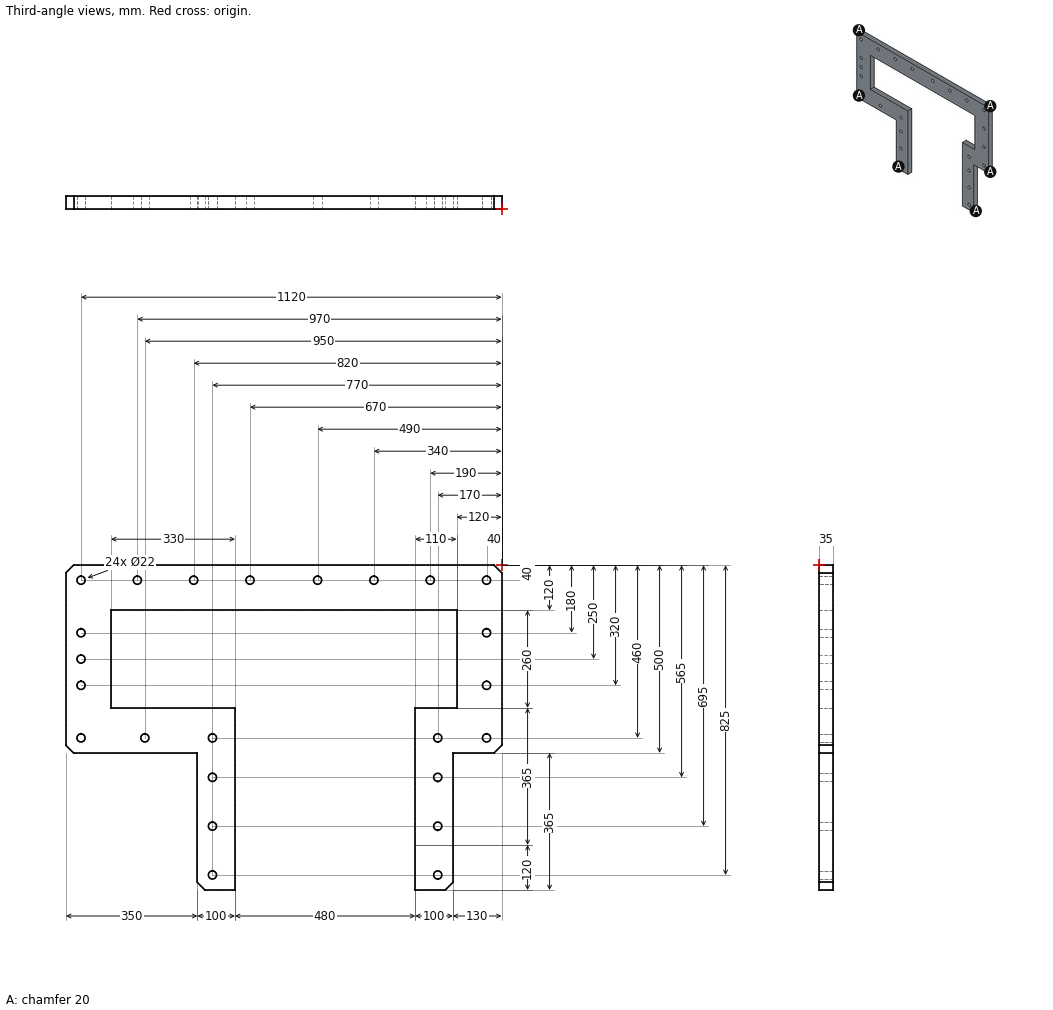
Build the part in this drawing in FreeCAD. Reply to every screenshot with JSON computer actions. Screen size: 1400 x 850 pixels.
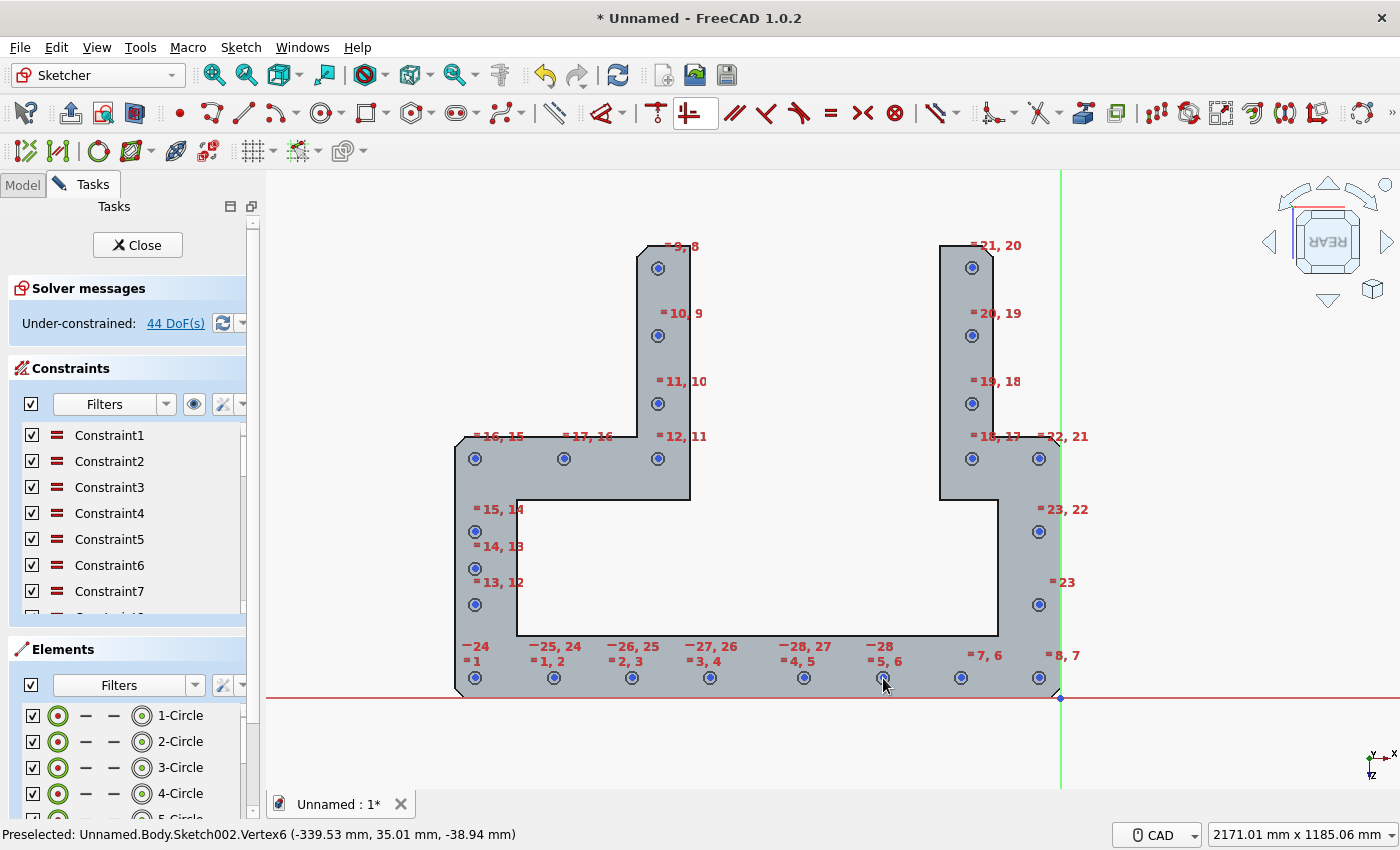
{"action": "left_click", "coordinate": [883, 678]}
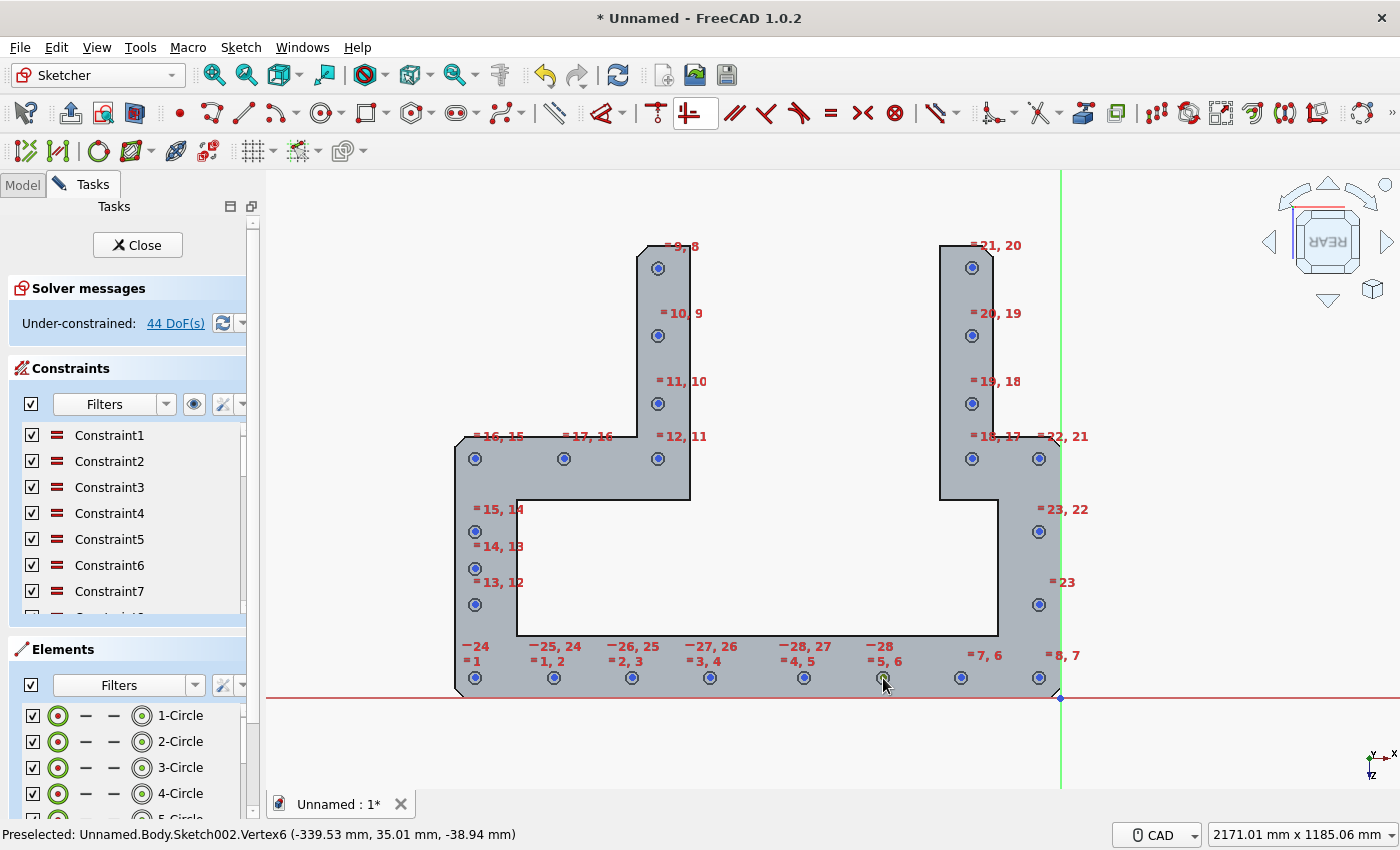
{"action": "left_click", "coordinate": [961, 678]}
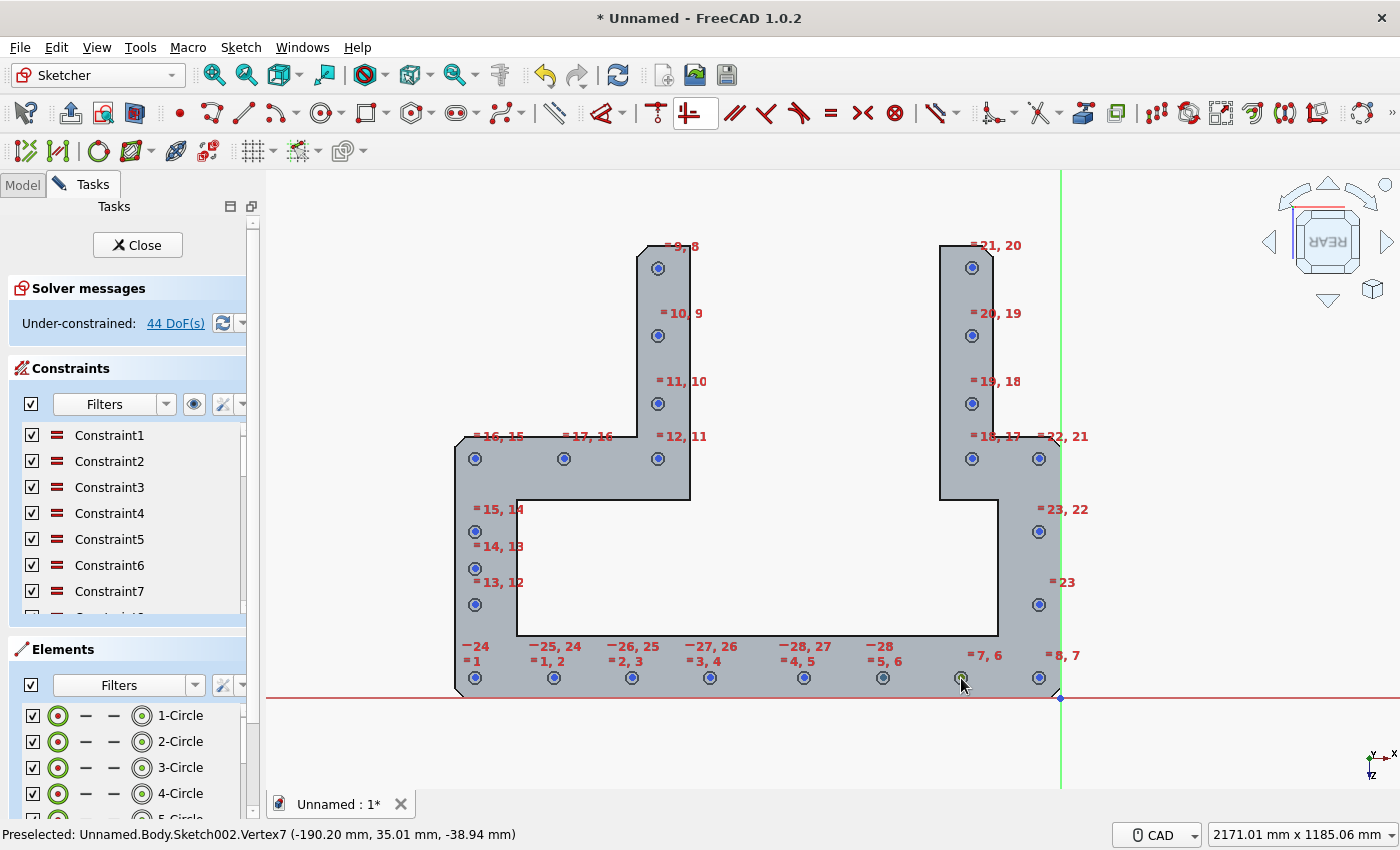
{"action": "left_click", "coordinate": [712, 114]}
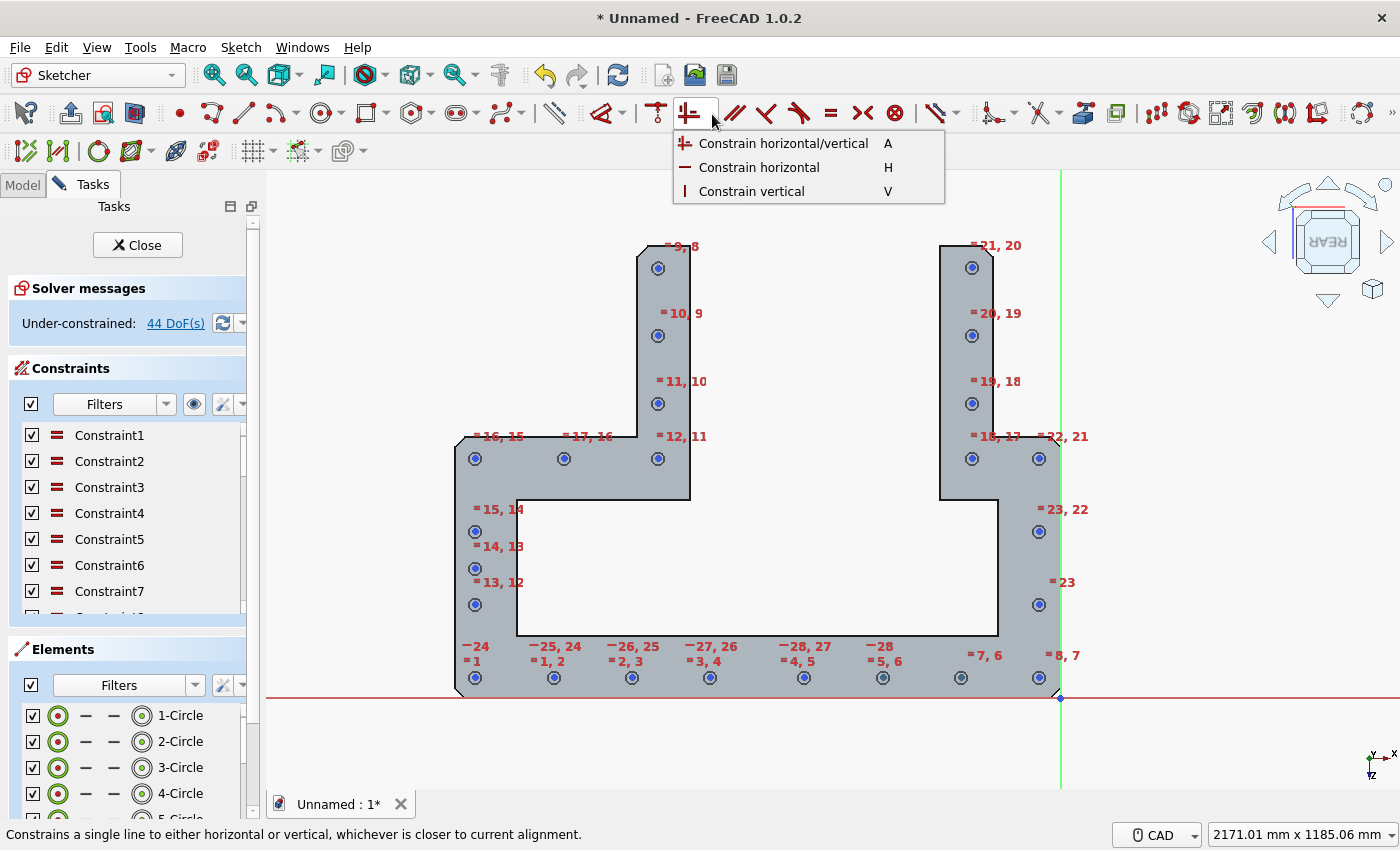
{"action": "left_click", "coordinate": [809, 167]}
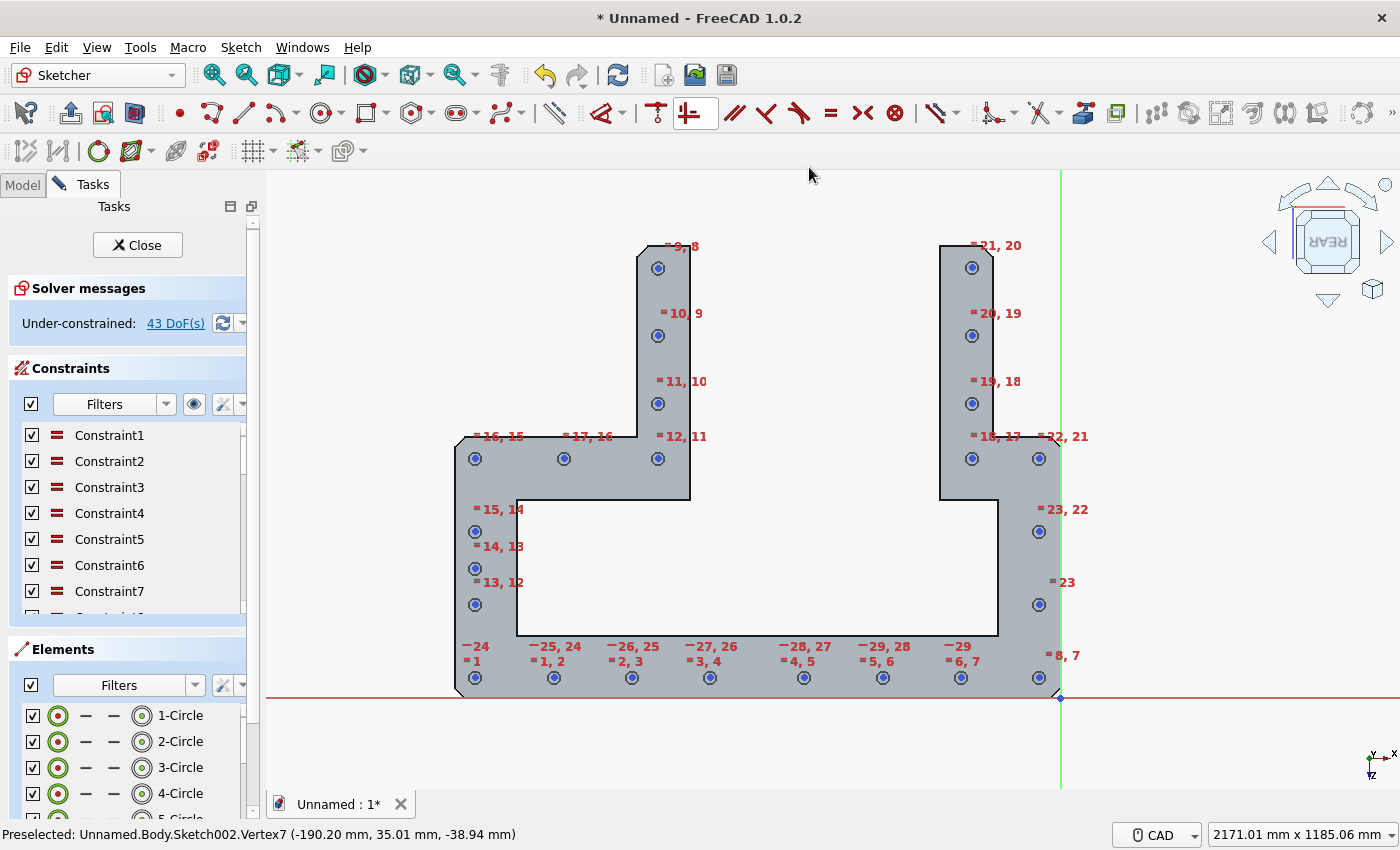
{"action": "left_click", "coordinate": [961, 678]}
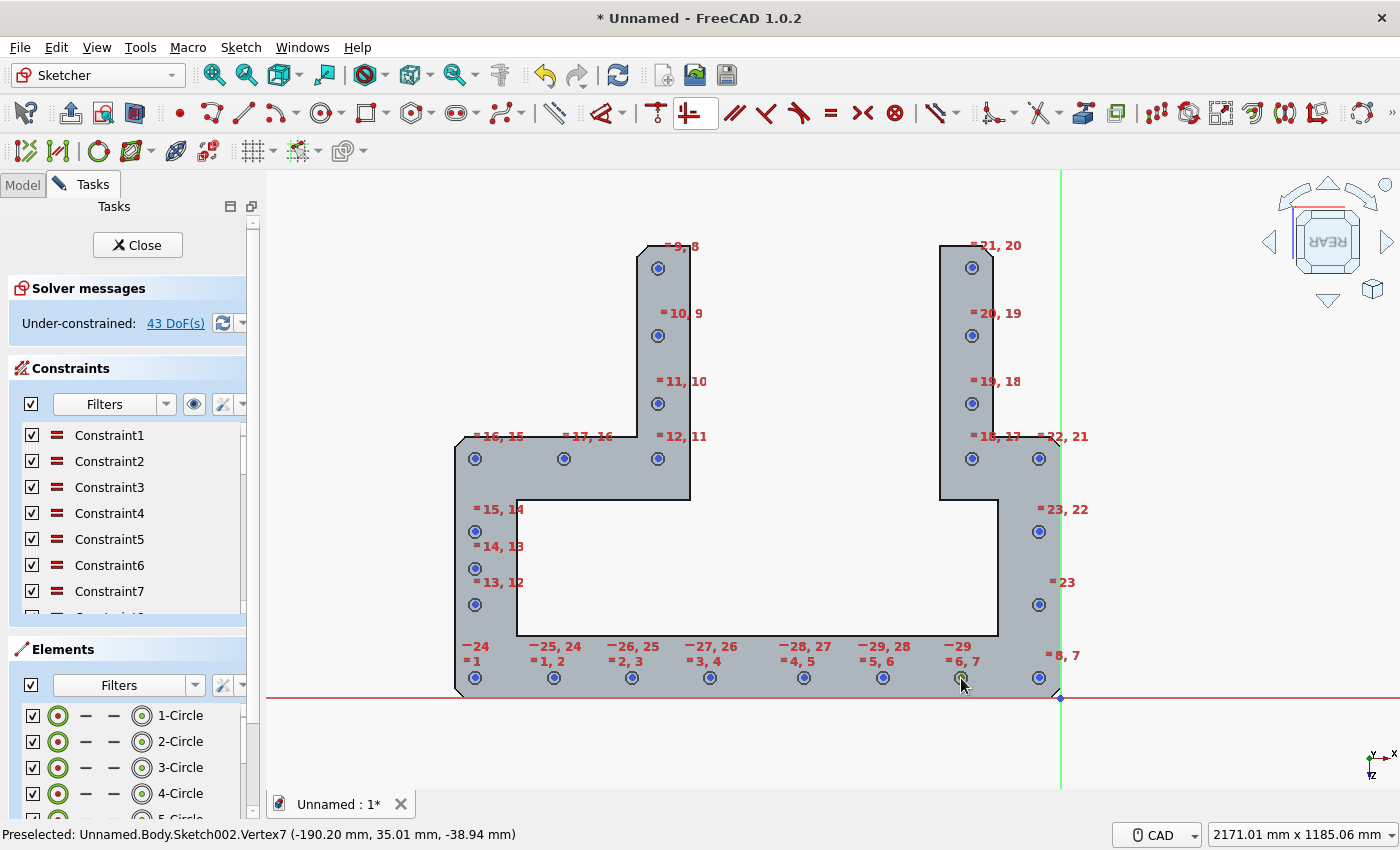
{"action": "left_click", "coordinate": [1039, 678]}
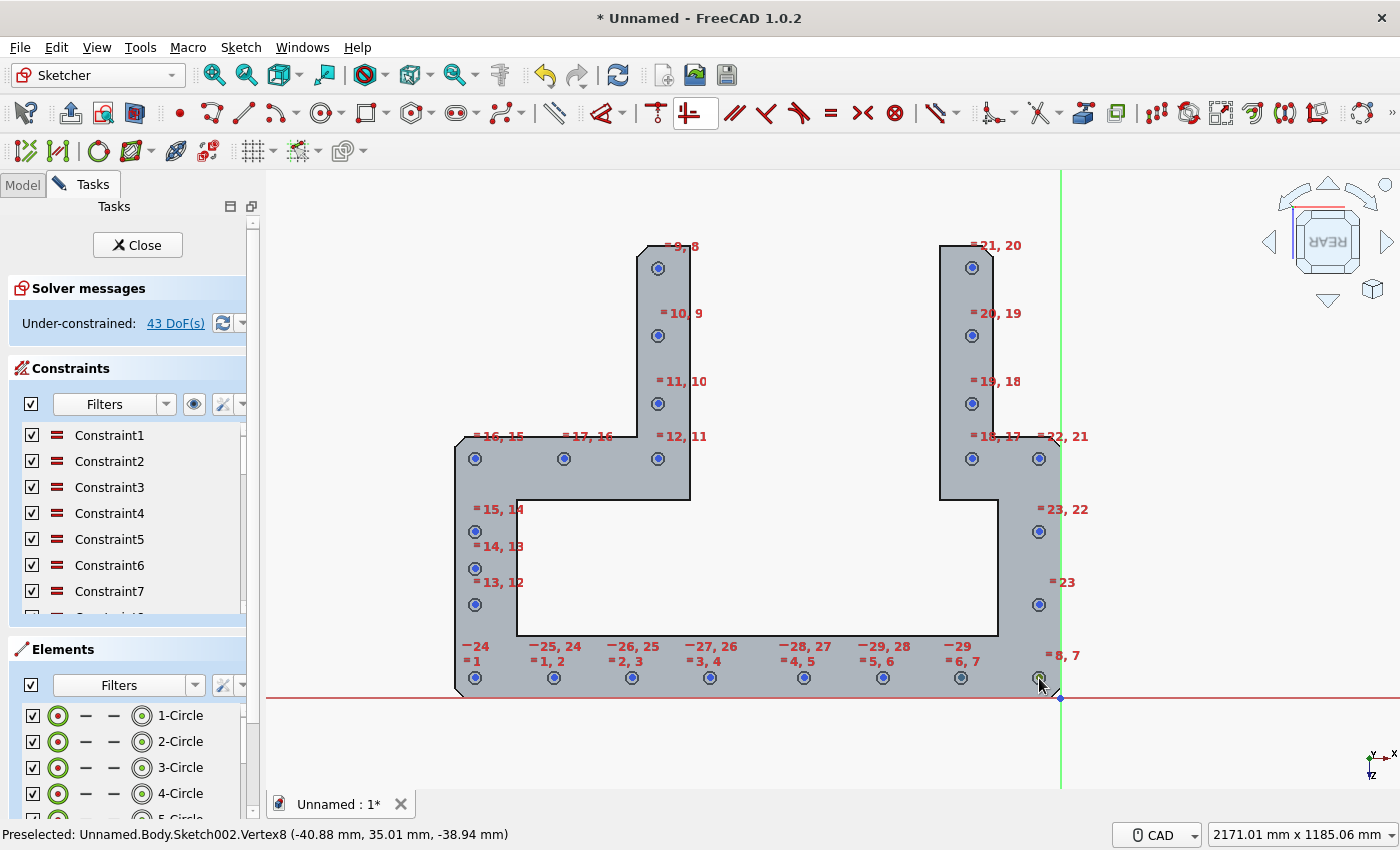
{"action": "key", "text": "h"}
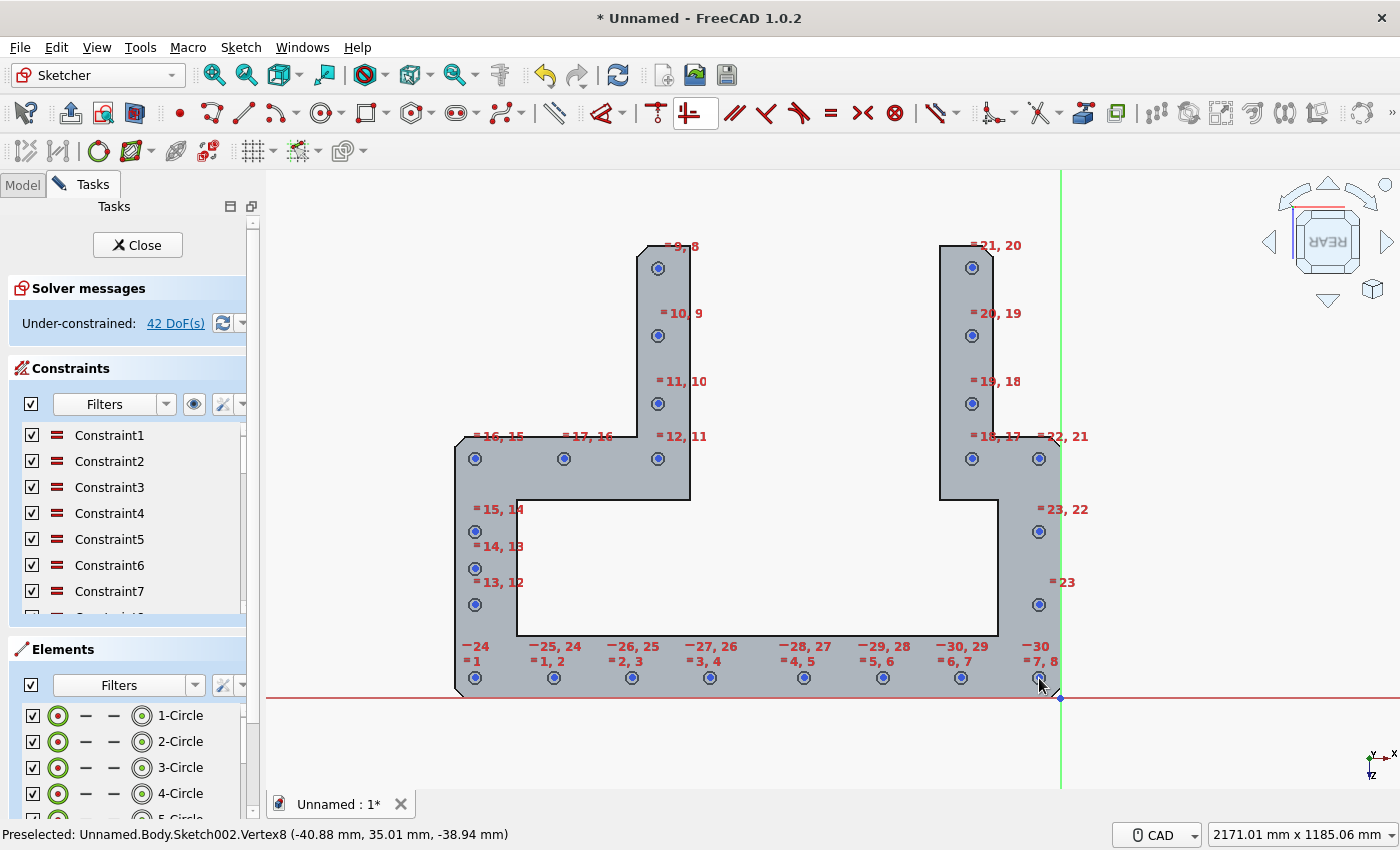
{"action": "left_click", "coordinate": [658, 269]}